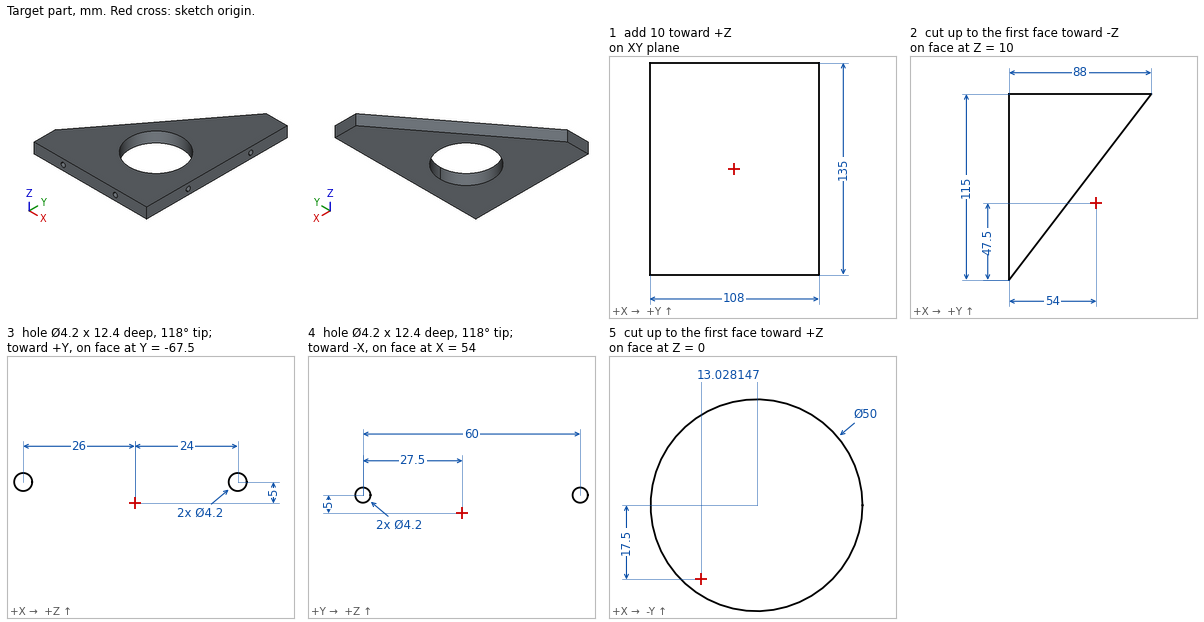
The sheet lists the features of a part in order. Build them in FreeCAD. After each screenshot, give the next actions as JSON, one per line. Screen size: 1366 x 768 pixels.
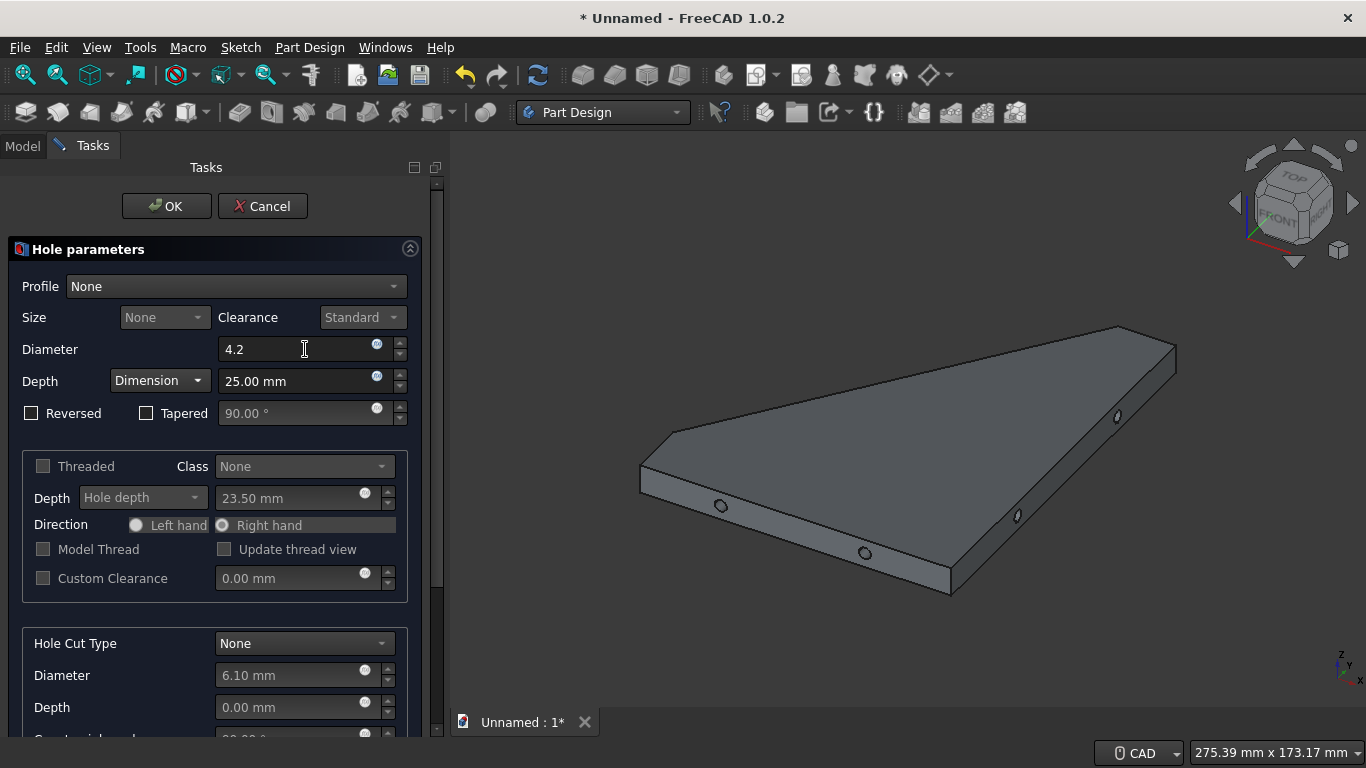
{"action": "triple_click", "coordinate": [305, 381]}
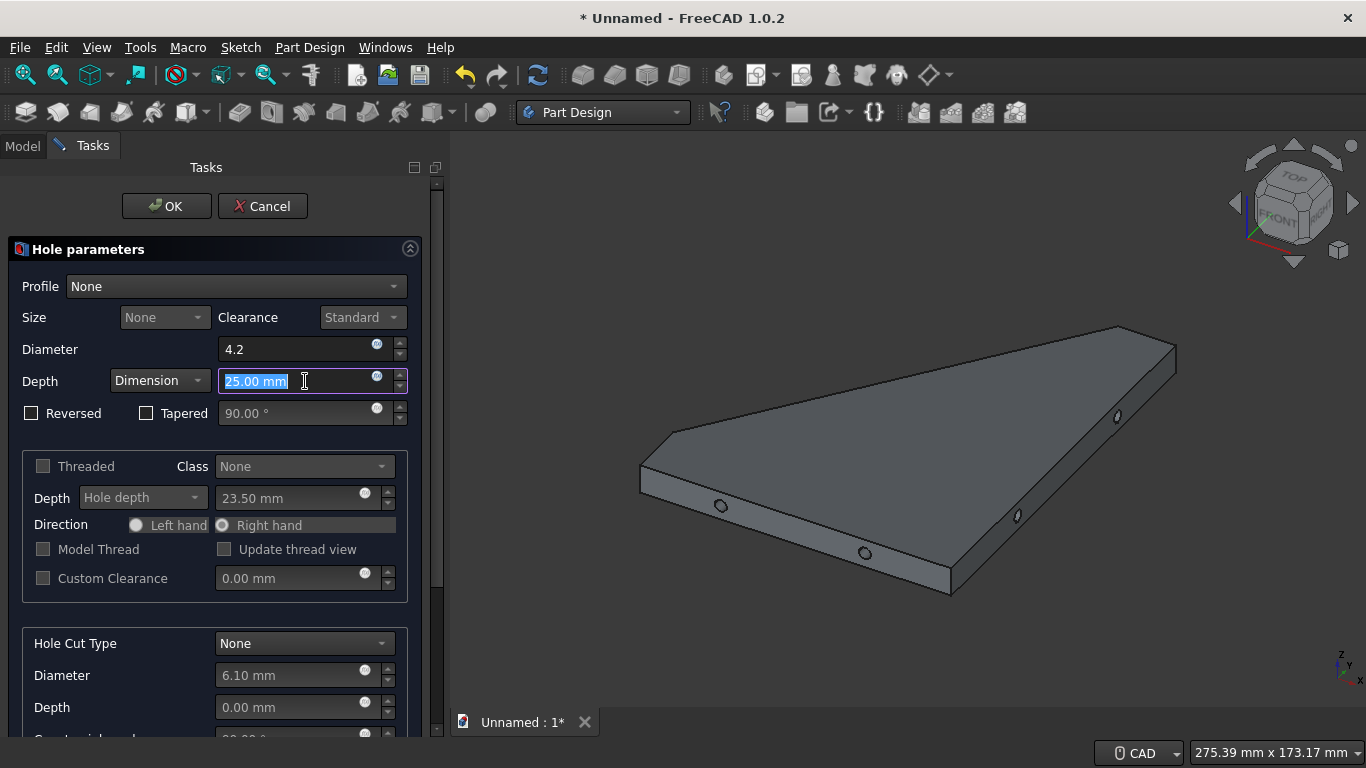
{"action": "type", "text": "12.4"}
{"action": "key", "text": "Tab"}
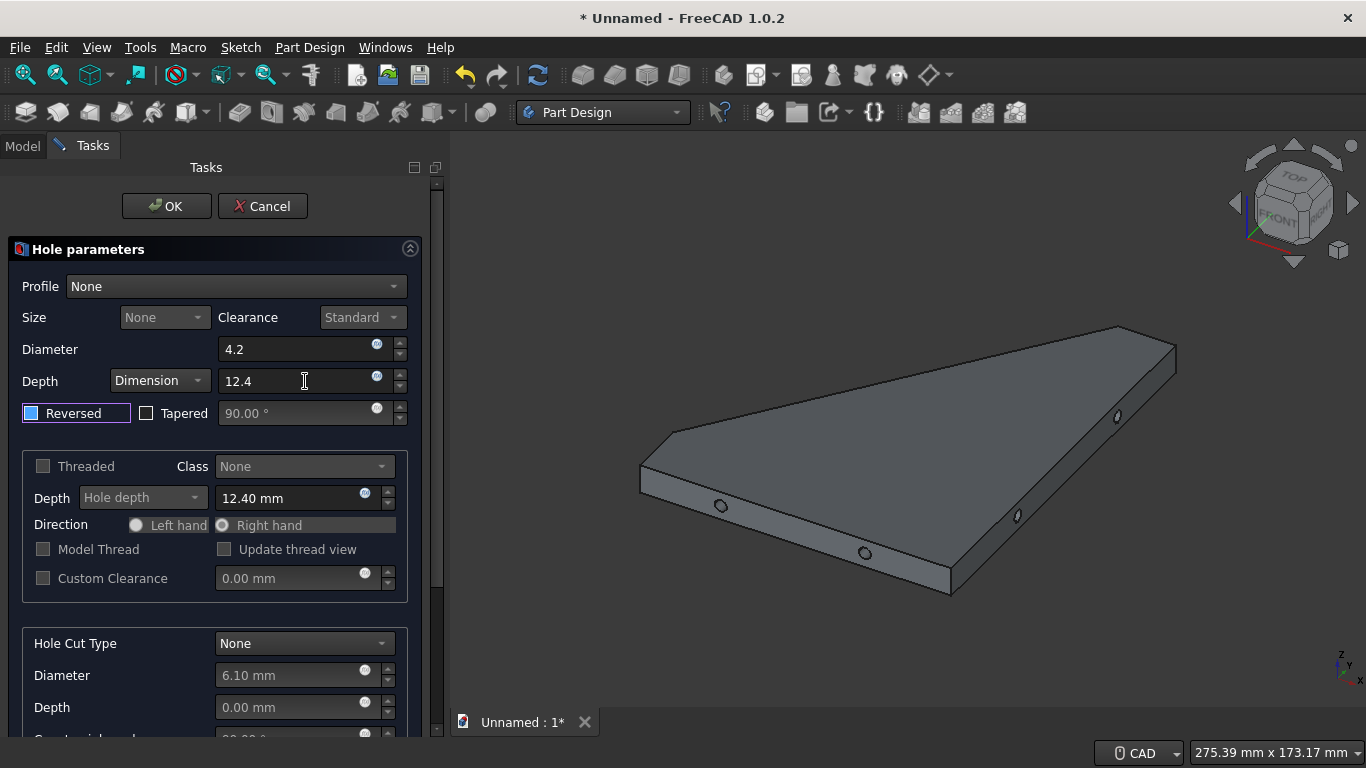
{"action": "left_click", "coordinate": [167, 206]}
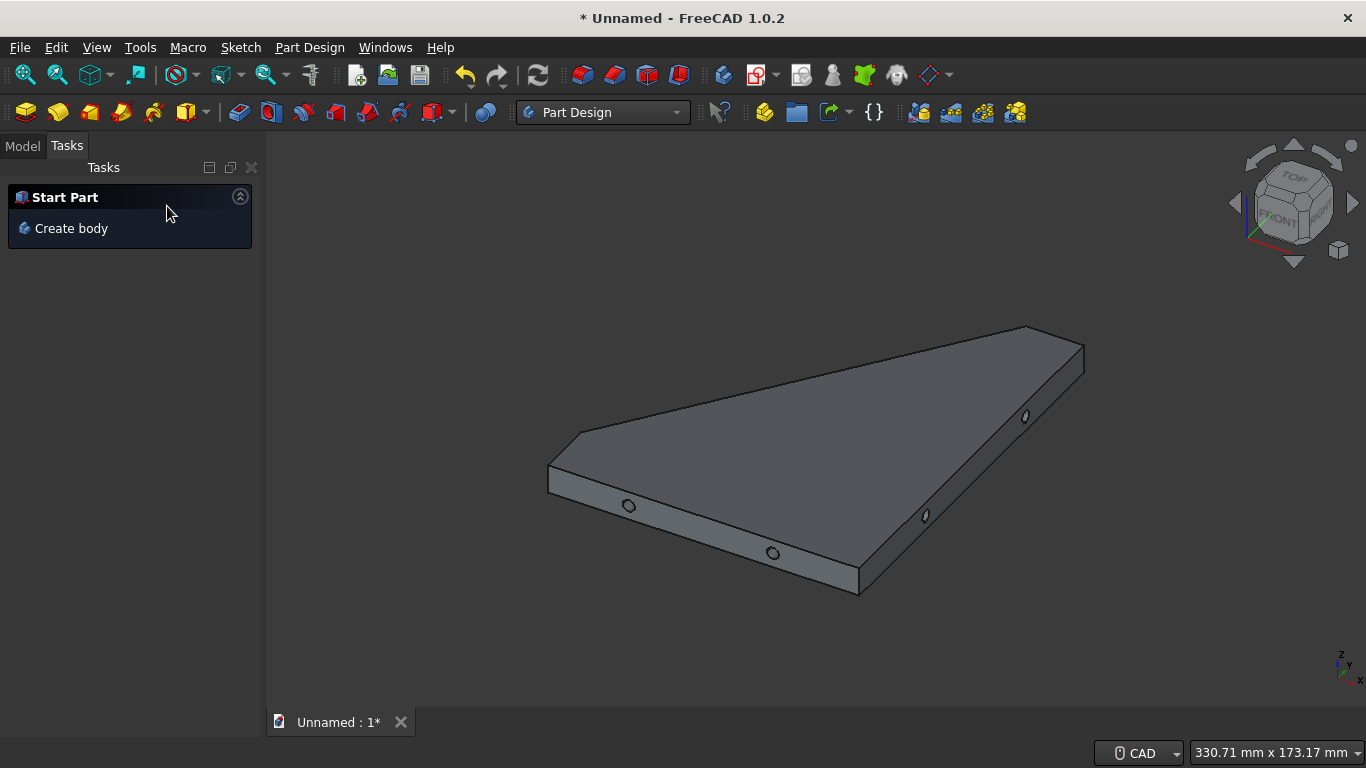
{"action": "key", "text": "5"}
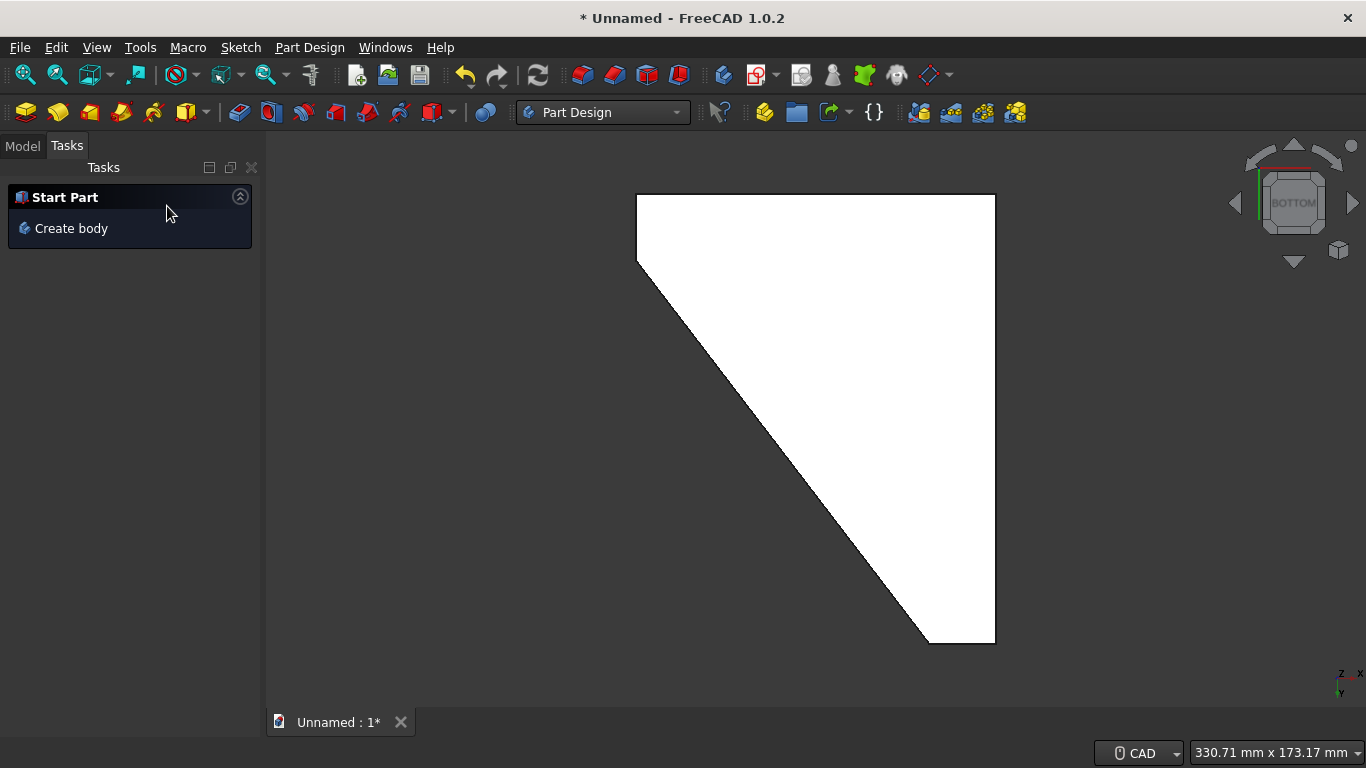
{"action": "left_click", "coordinate": [867, 354]}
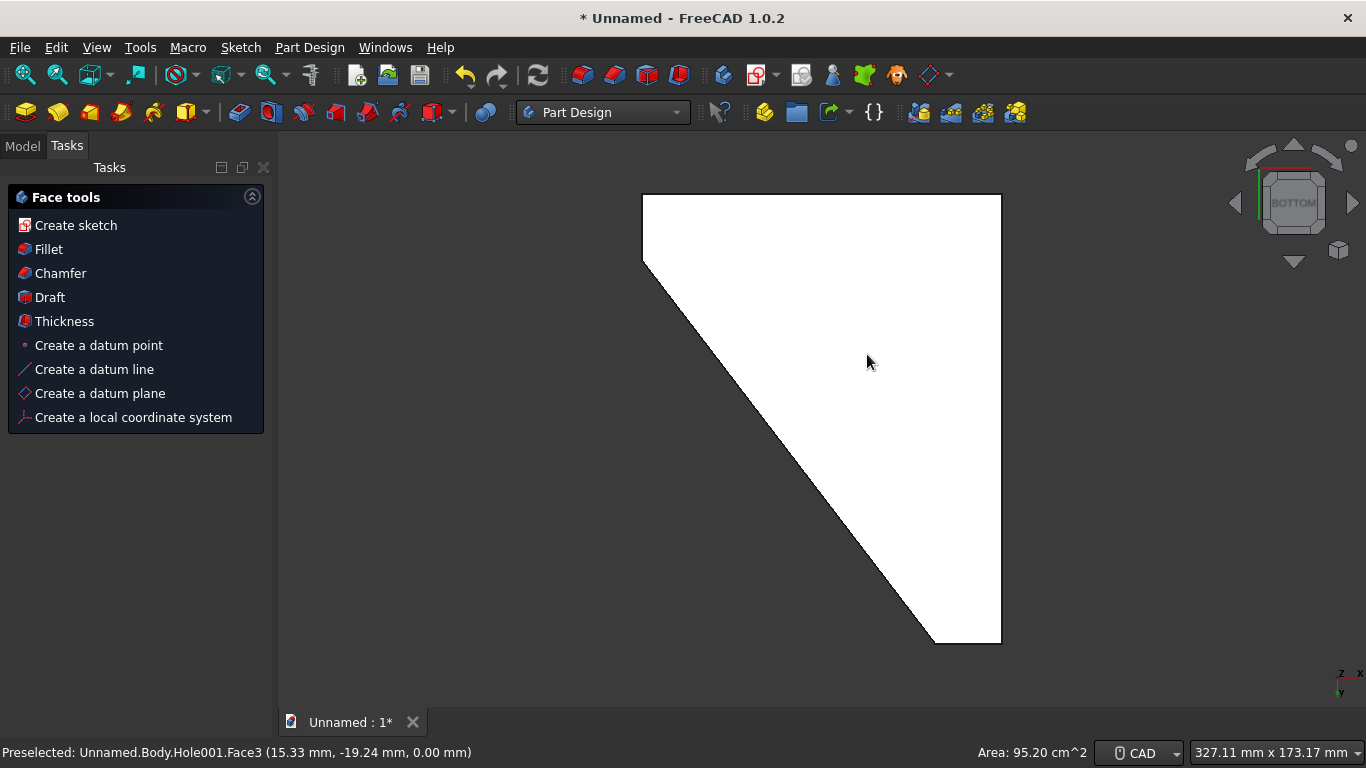
{"action": "left_click", "coordinate": [756, 76]}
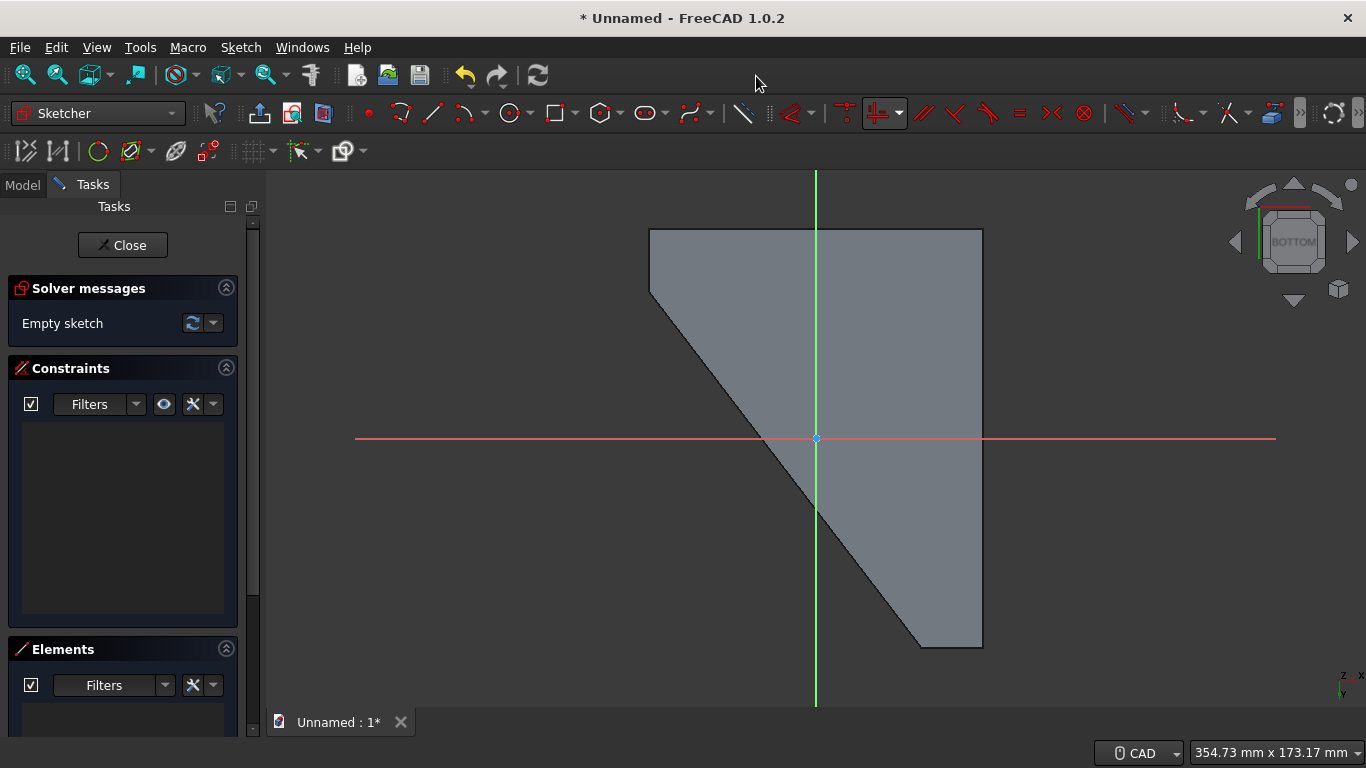
{"action": "scroll", "coordinate": [945, 340], "scroll_direction": "up", "scroll_amount": 4}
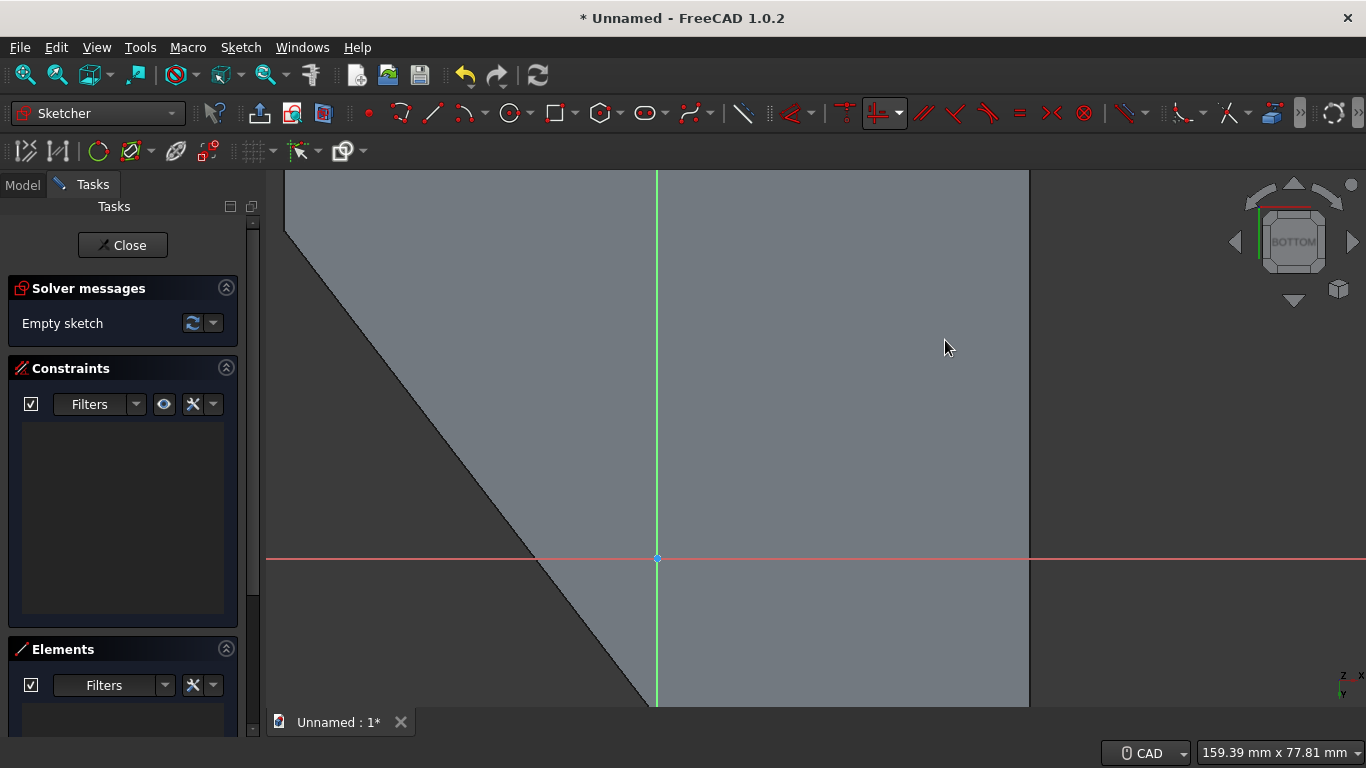
{"action": "left_click", "coordinate": [510, 114]}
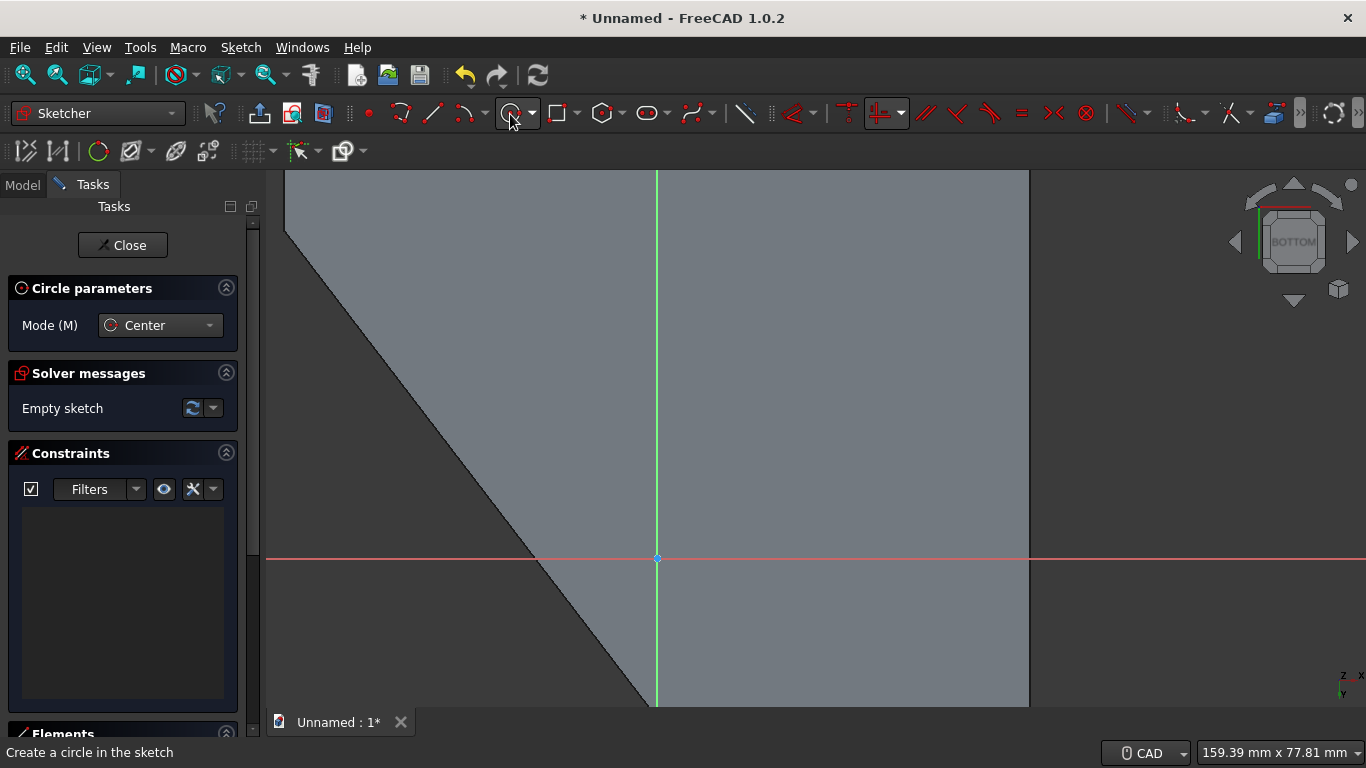
{"action": "left_click", "coordinate": [747, 438]}
{"action": "mouse_move", "coordinate": [869, 316]}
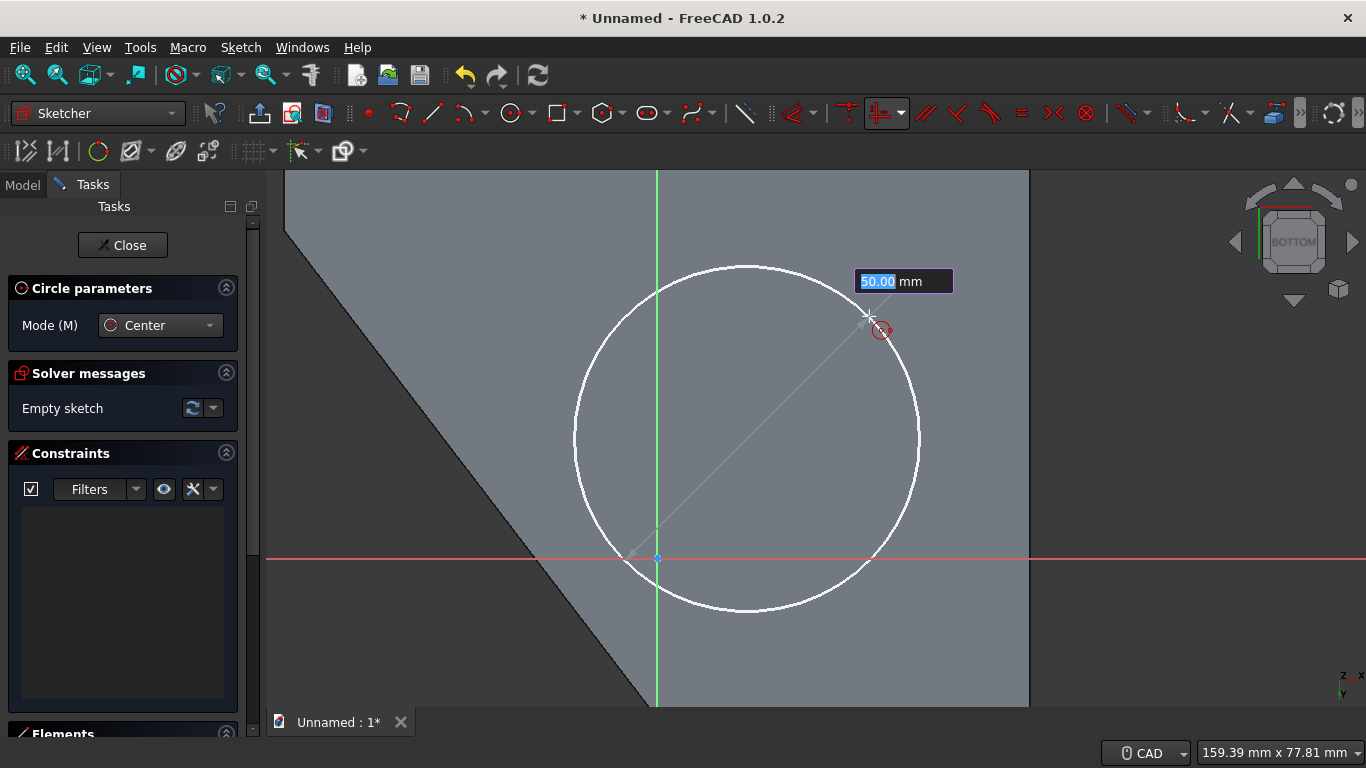
{"action": "type", "text": "50"}
{"action": "key", "text": "Return"}
{"action": "key", "text": "Escape"}